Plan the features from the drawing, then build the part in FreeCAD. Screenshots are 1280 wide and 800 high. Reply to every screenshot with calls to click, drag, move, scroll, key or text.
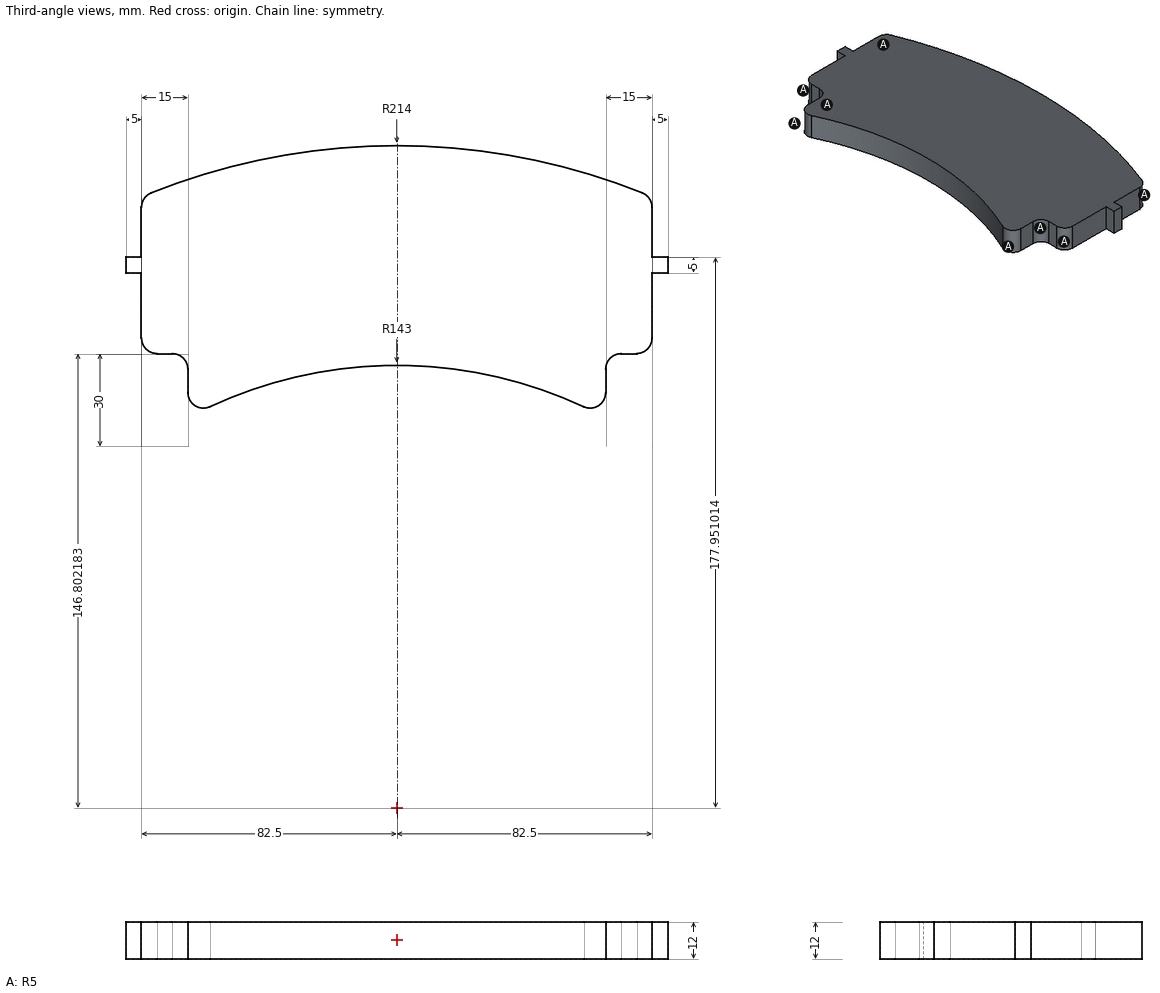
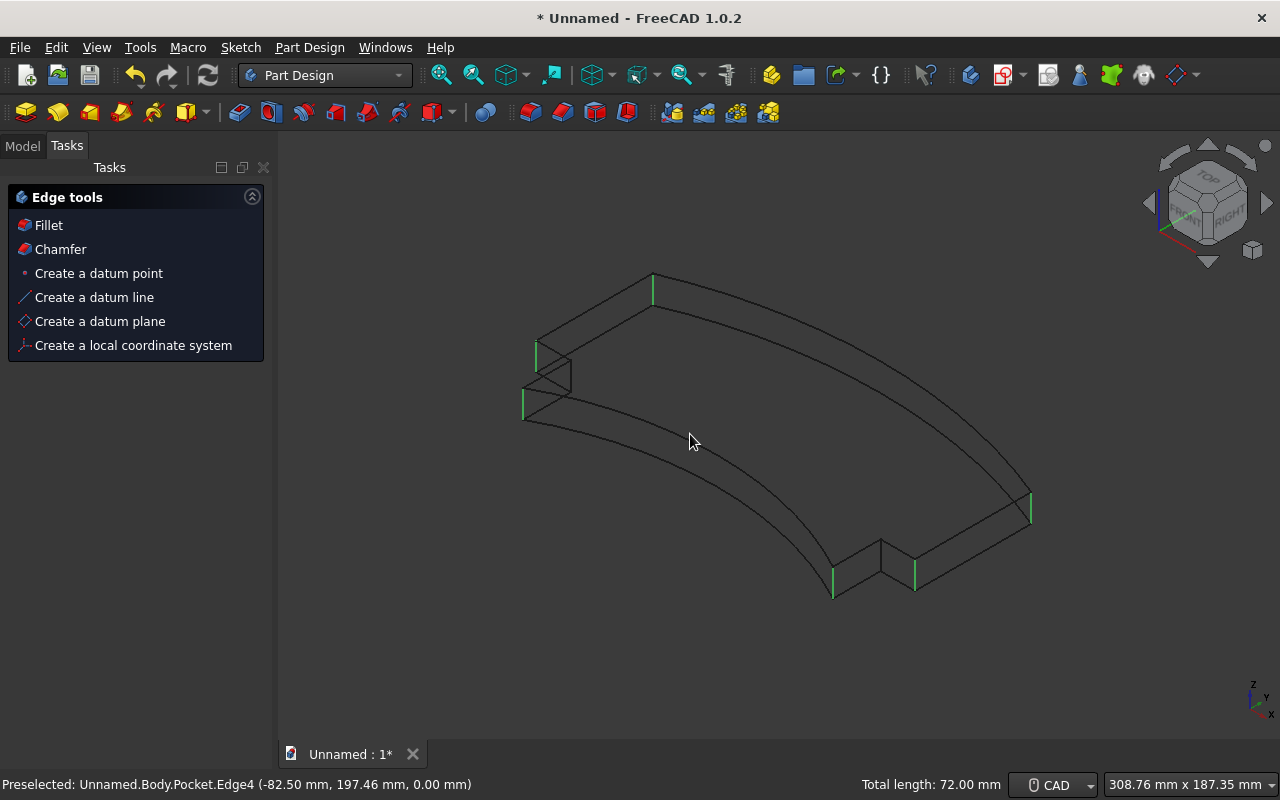
click(571, 375, ctrl)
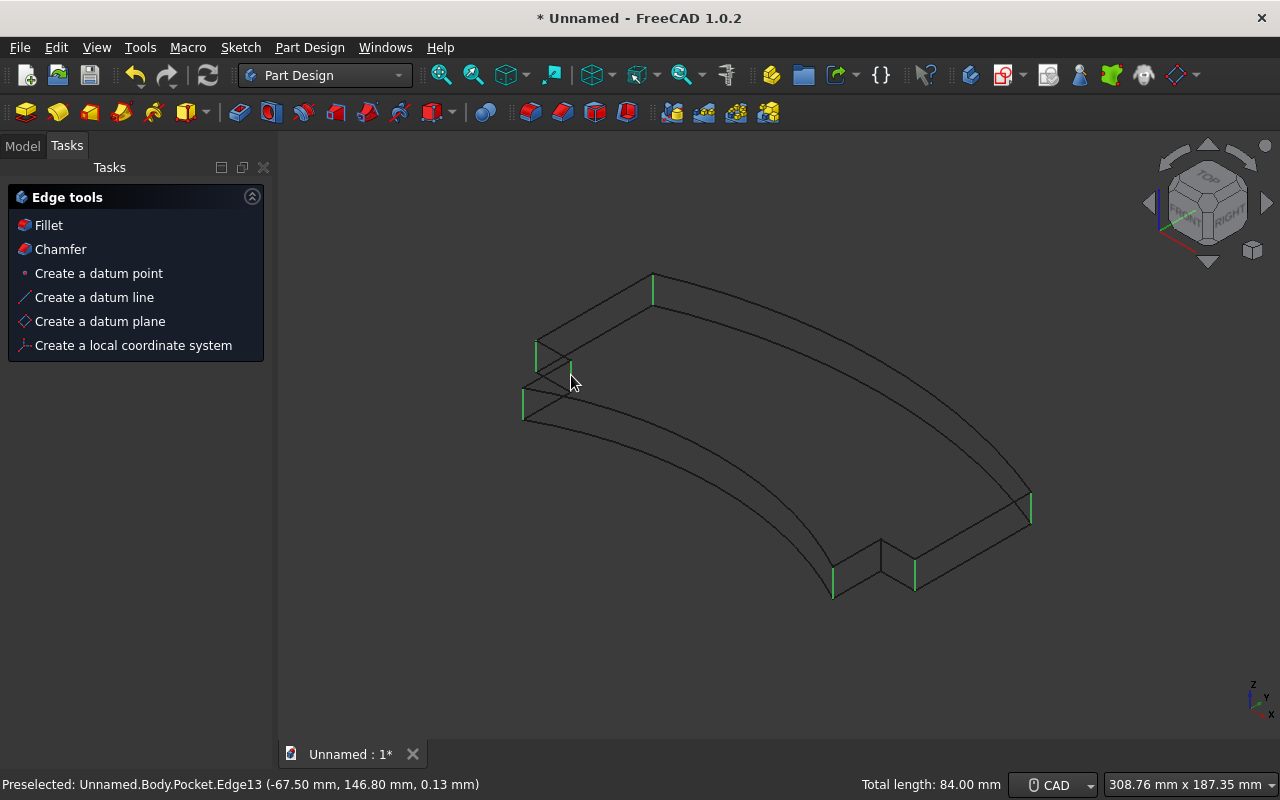
click(881, 554, ctrl)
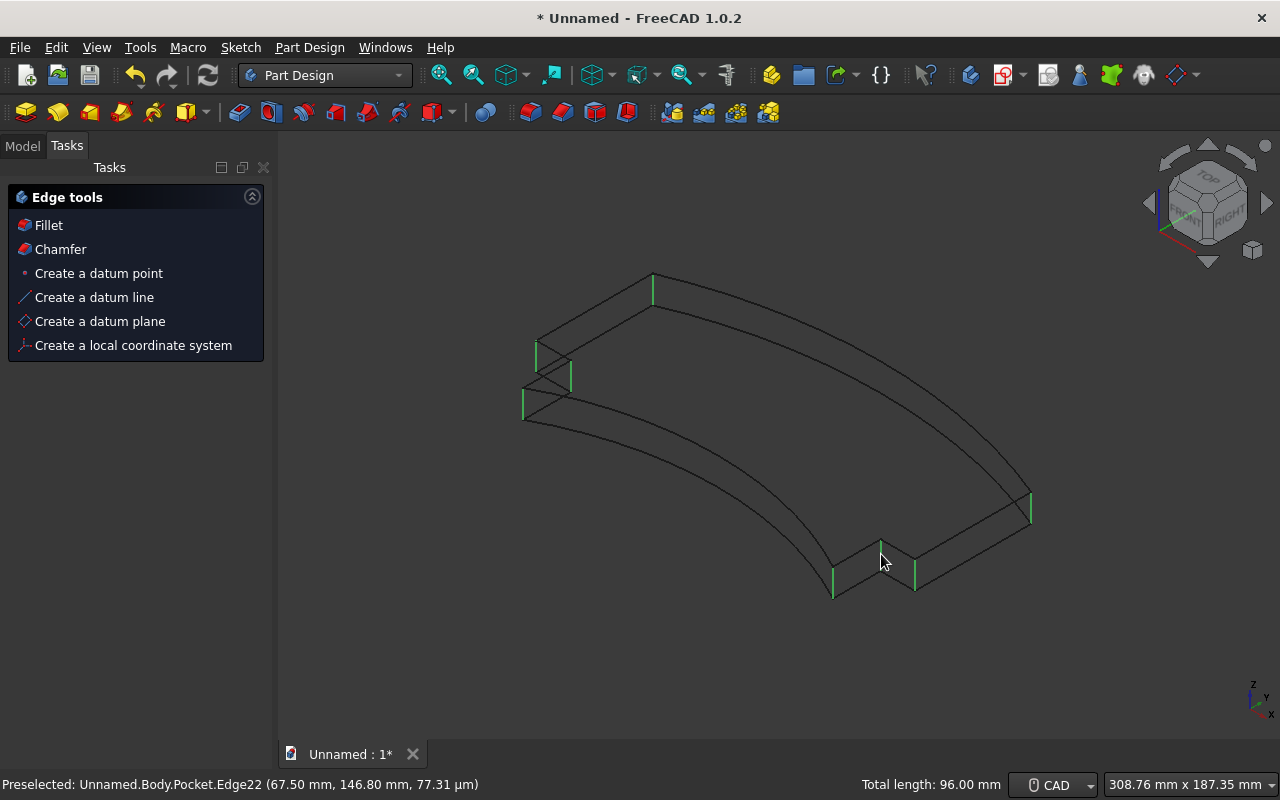
key(v)
key(1)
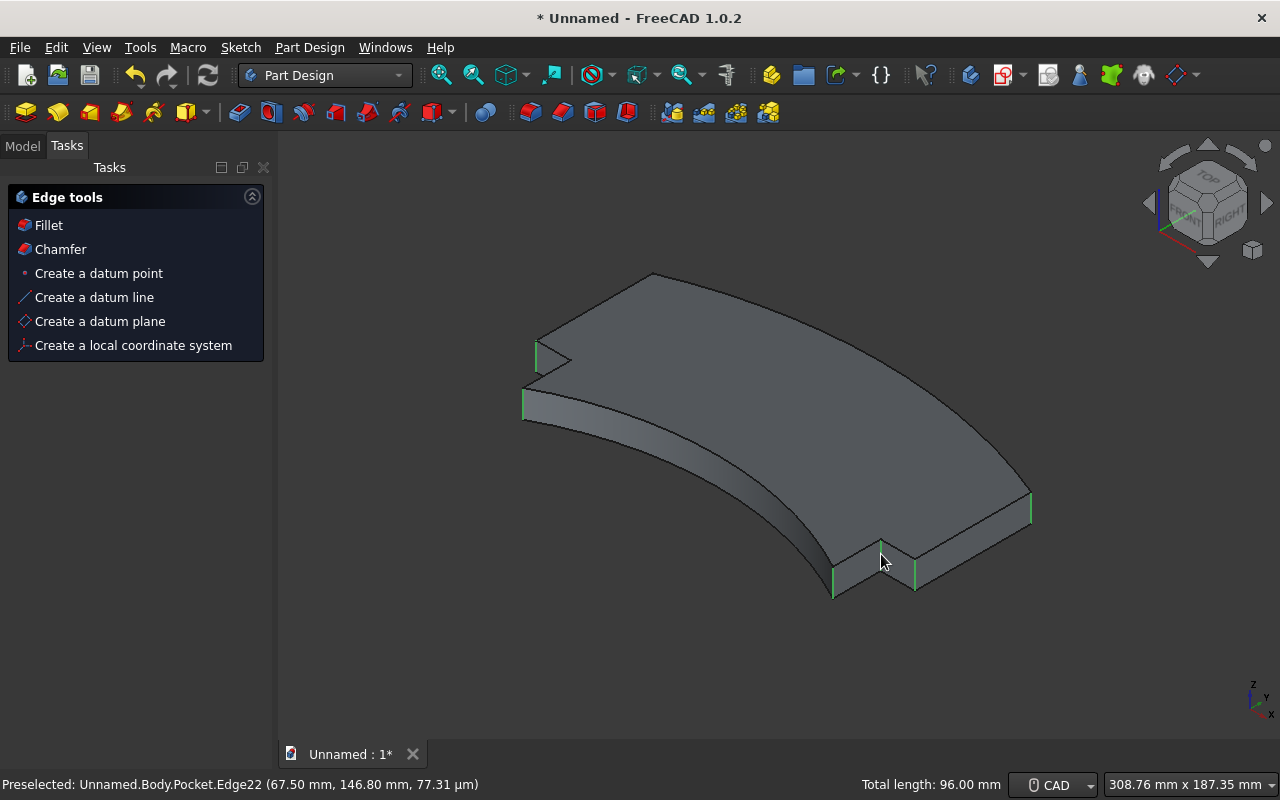
click(532, 112)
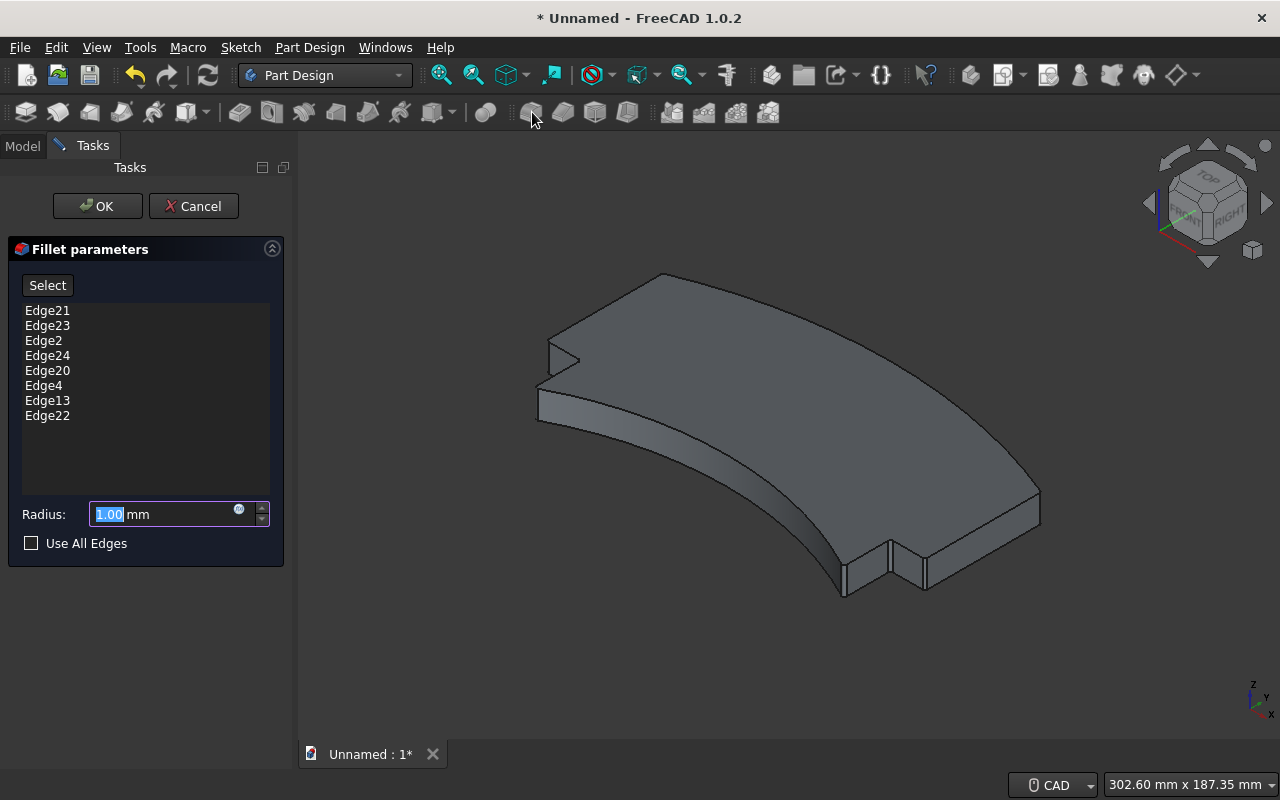
text(5)
key(Tab)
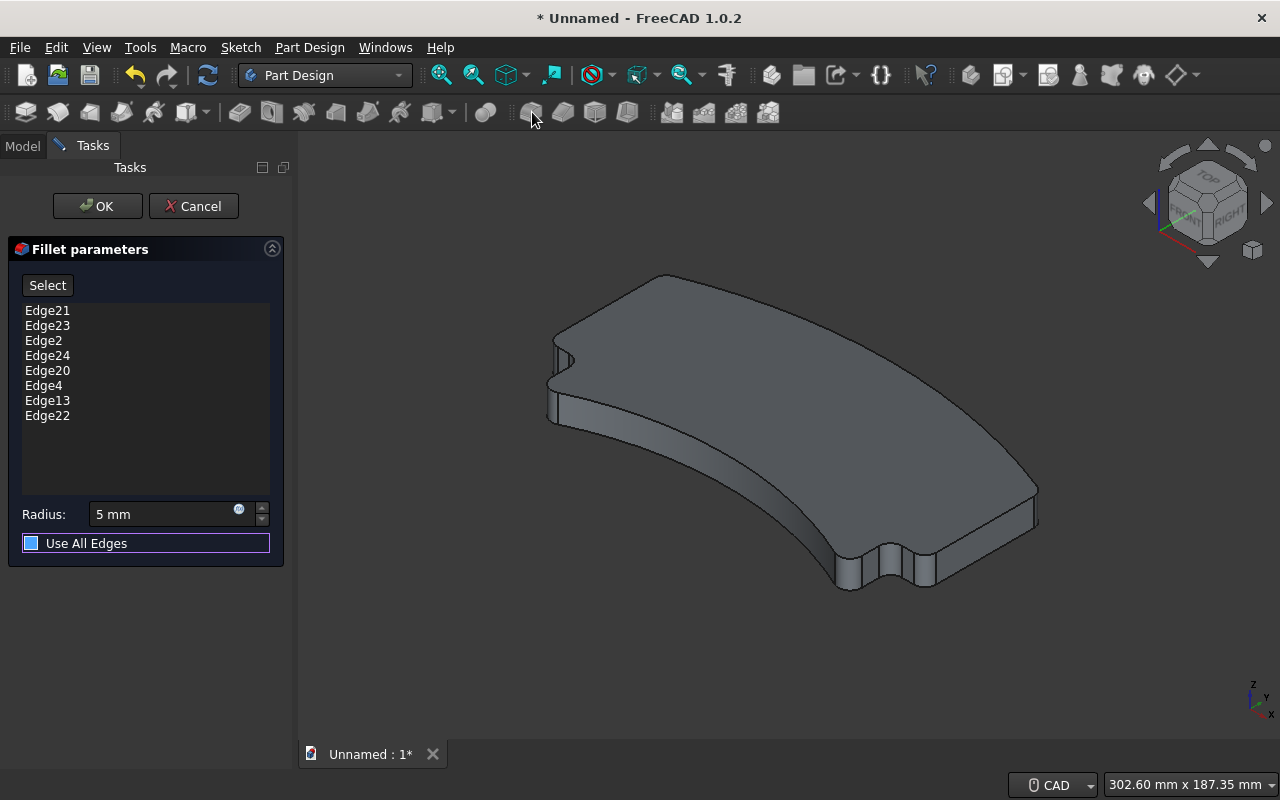
click(98, 206)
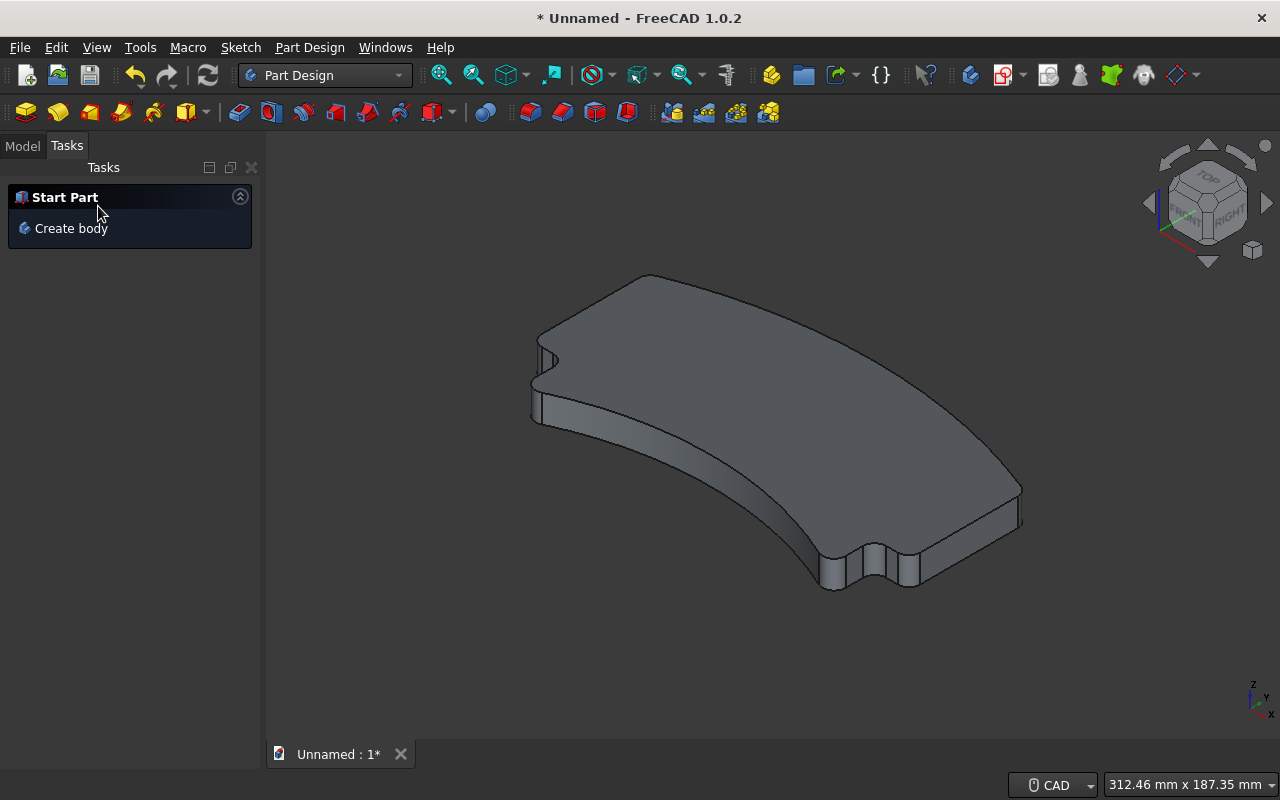
click(885, 479)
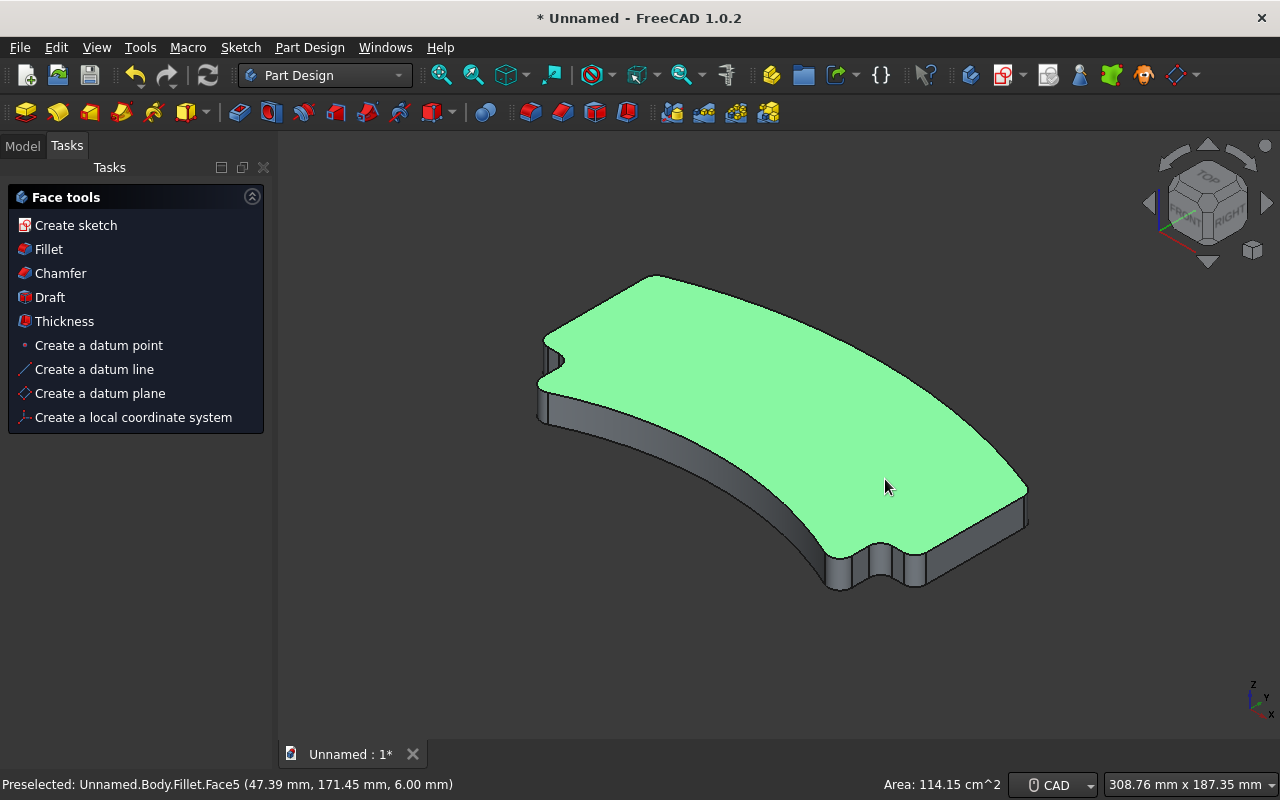
click(1004, 76)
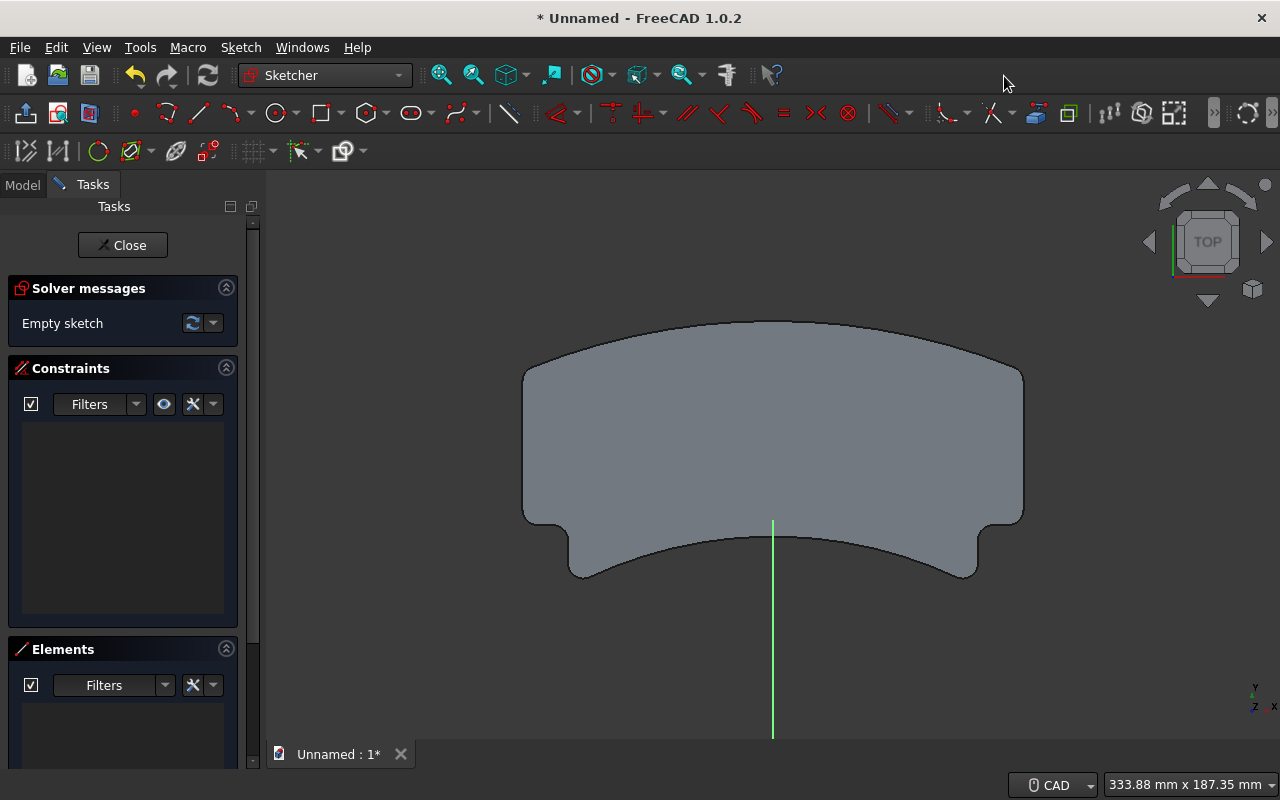
scroll(621, 198, down, 3)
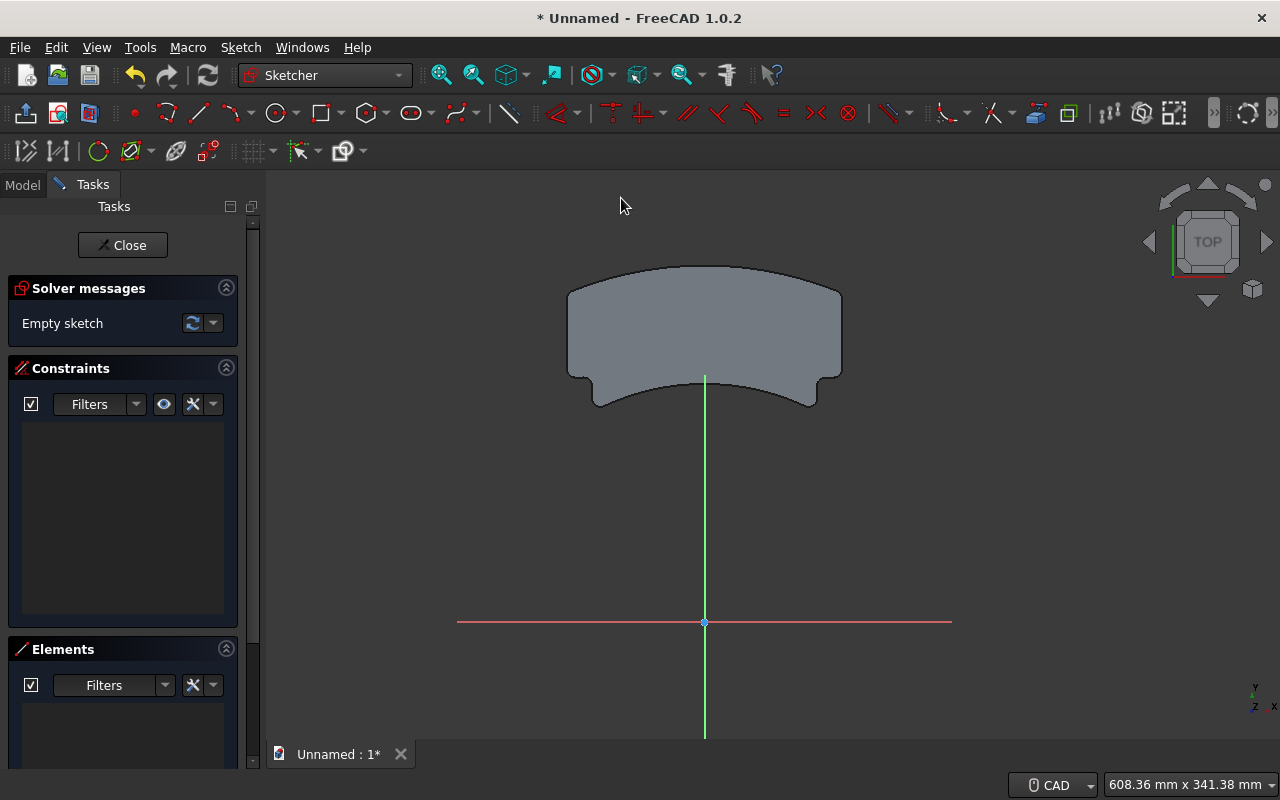
click(322, 114)